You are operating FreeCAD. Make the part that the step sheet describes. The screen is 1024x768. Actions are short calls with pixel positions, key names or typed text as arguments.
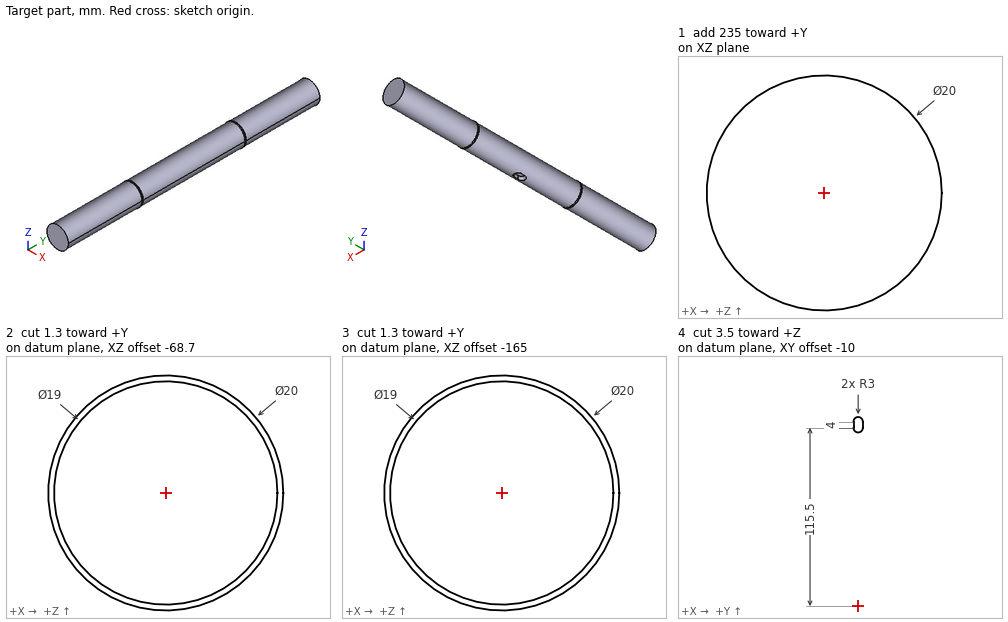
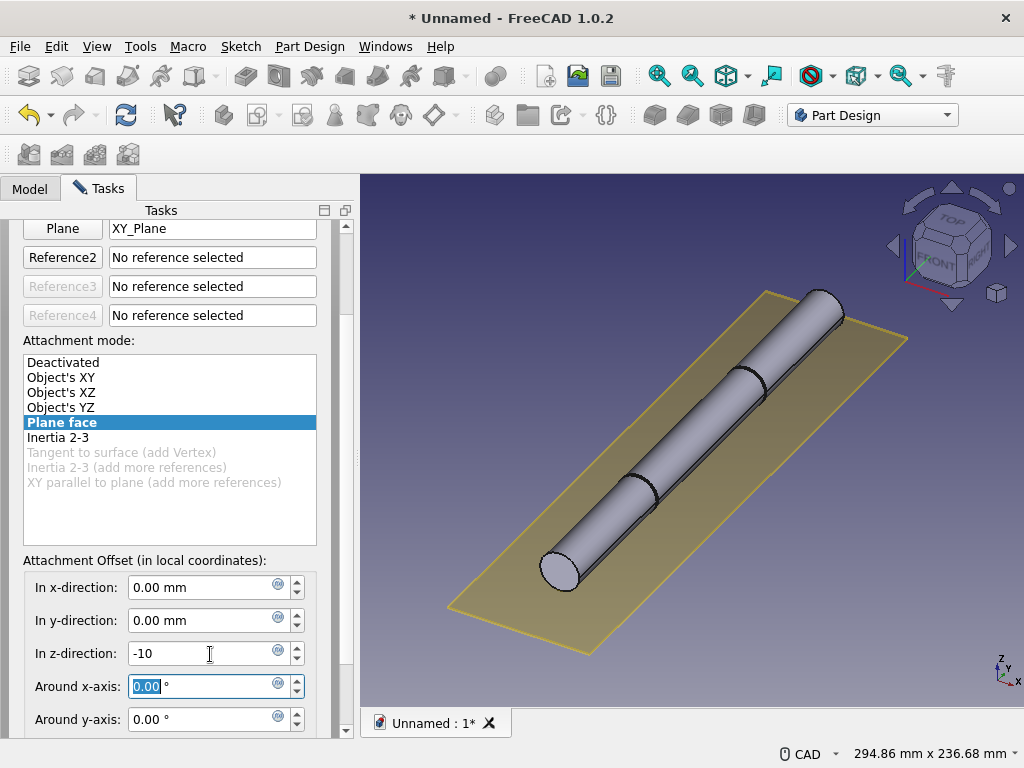
scroll(346, 479, up, 3)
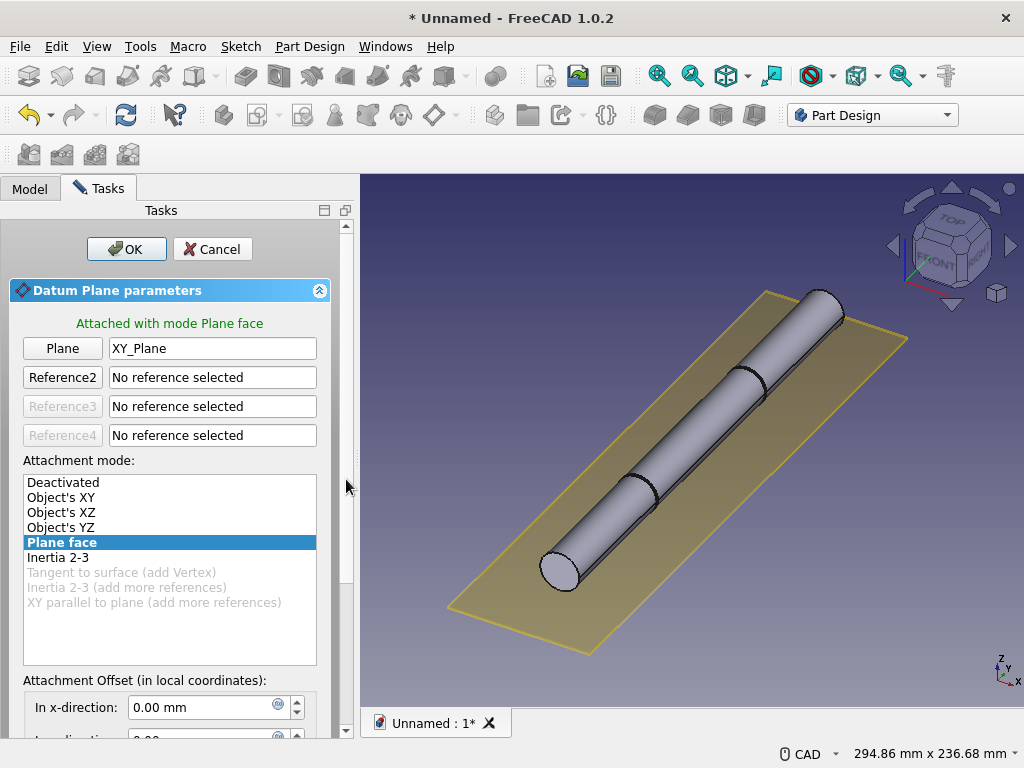
click(127, 249)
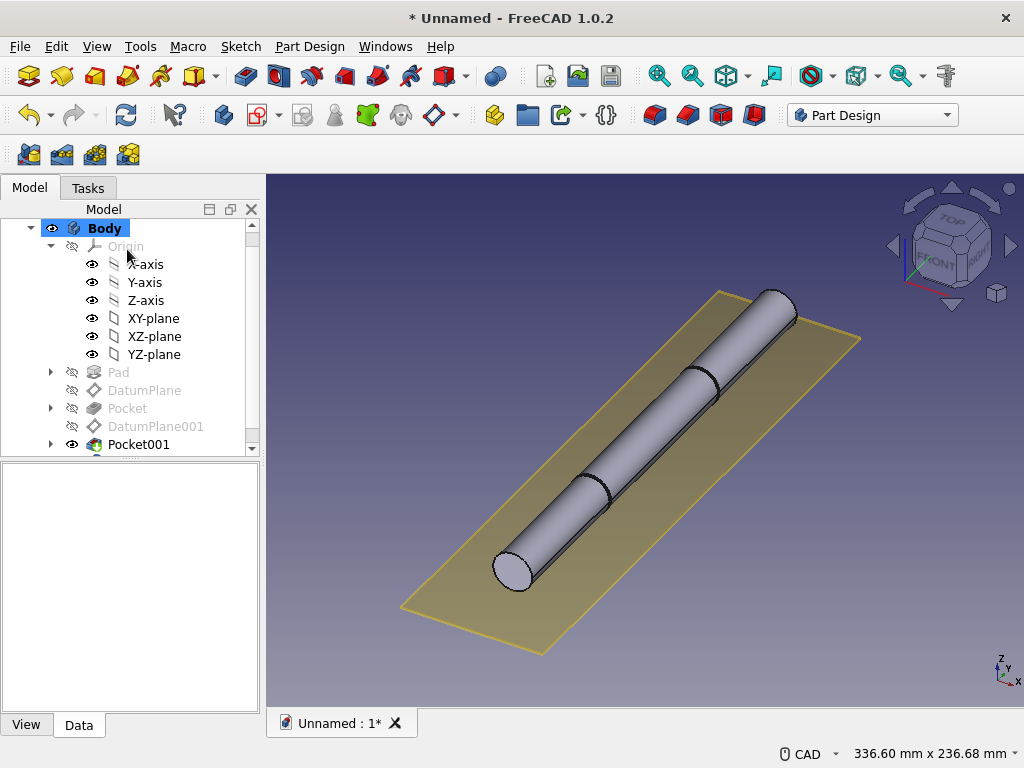
scroll(121, 332, down, 3)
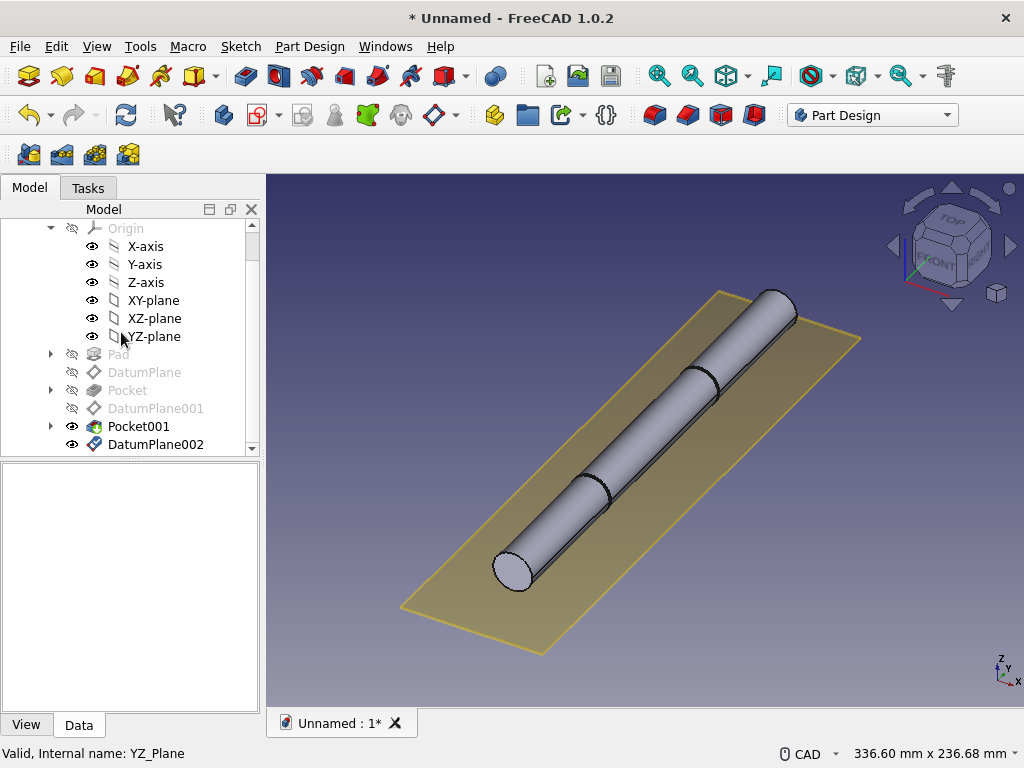
click(117, 444)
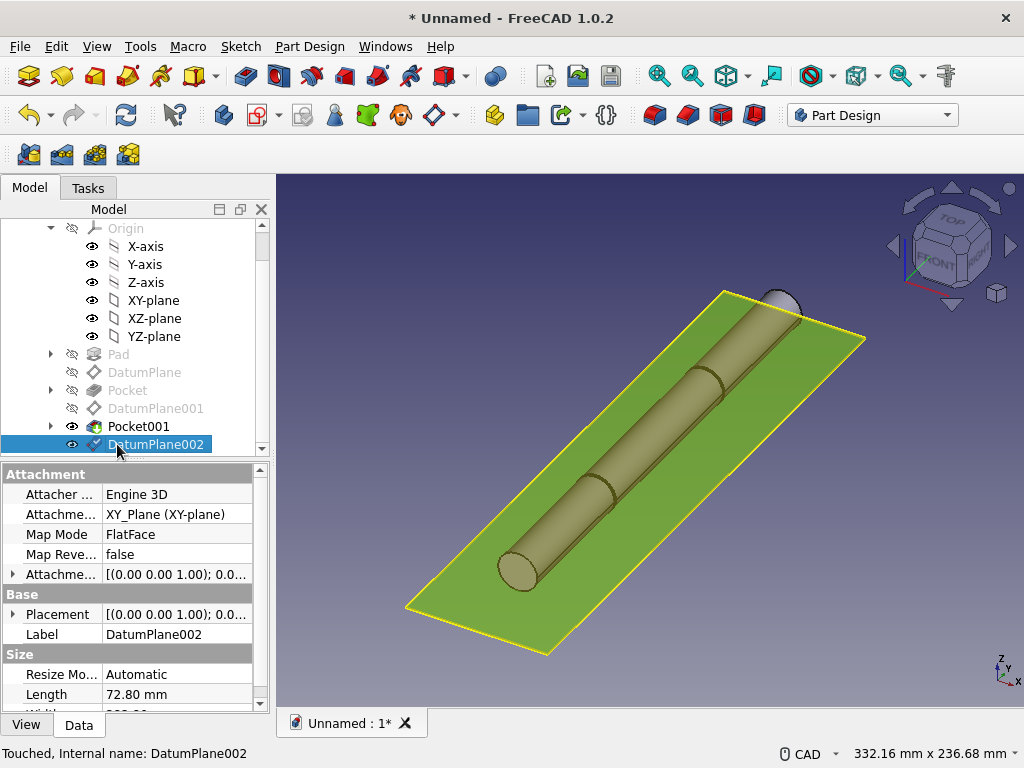
click(256, 116)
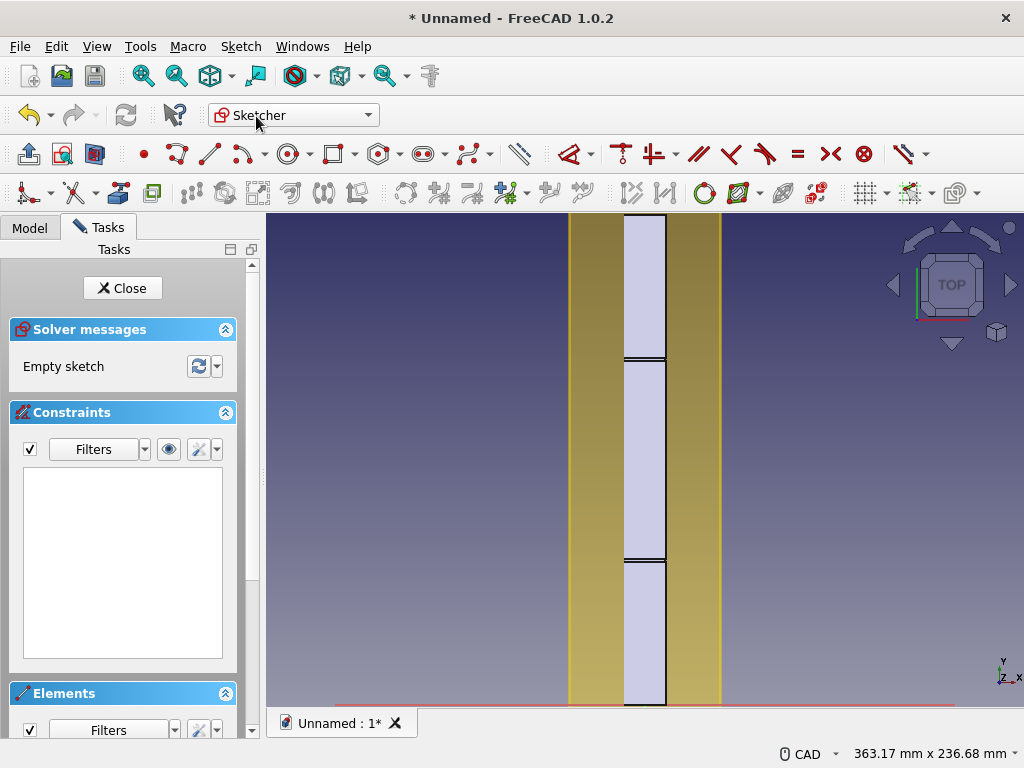
key(q)
key(s)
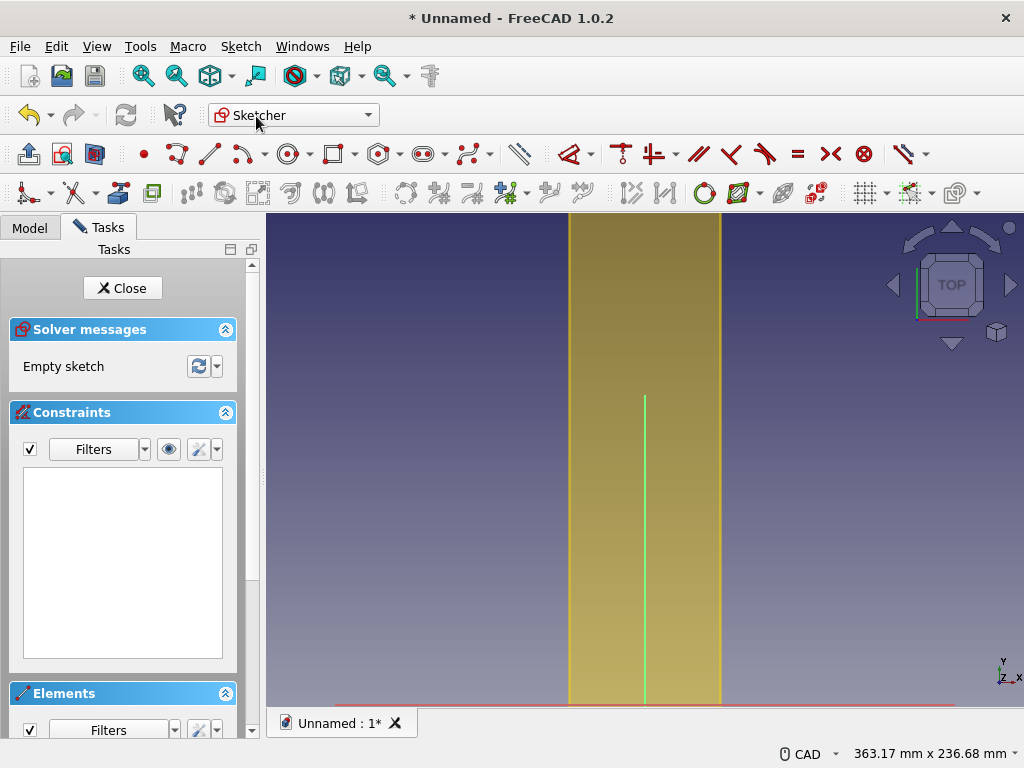
scroll(650, 460, up, 13)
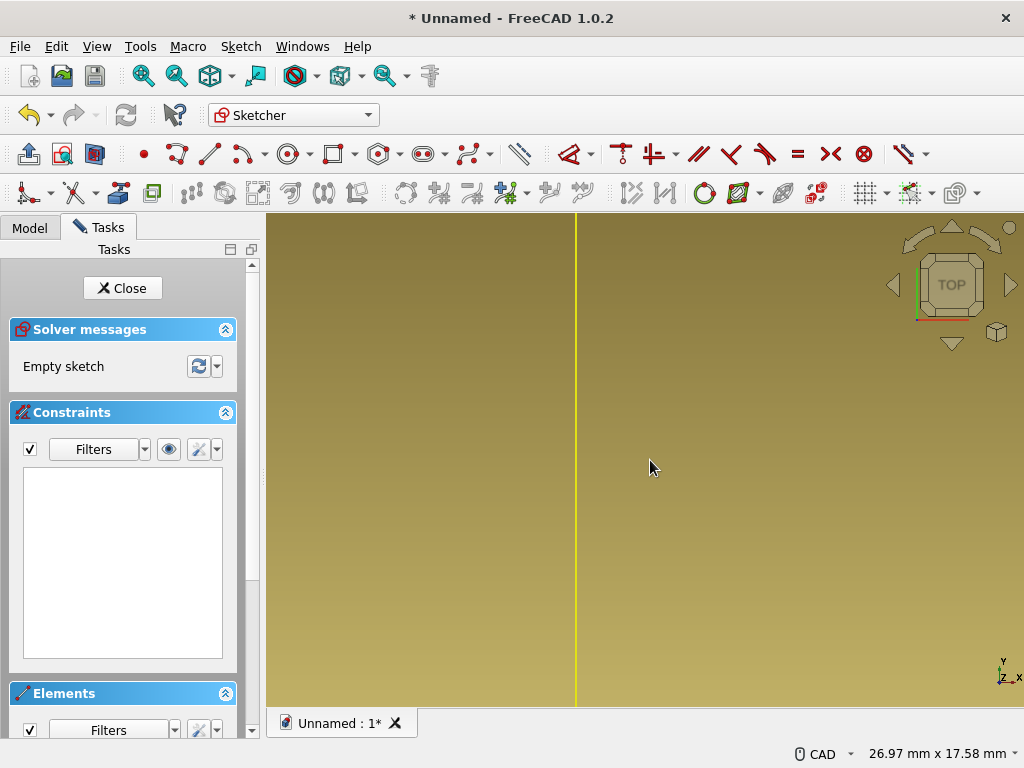
click(422, 154)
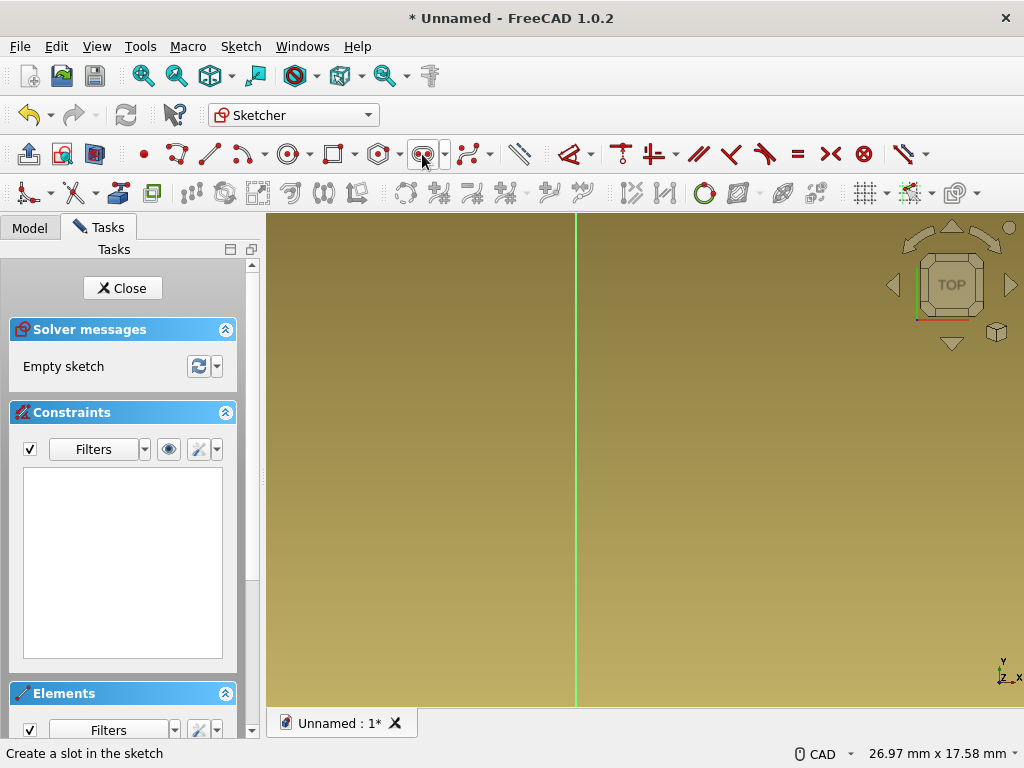
click(576, 510)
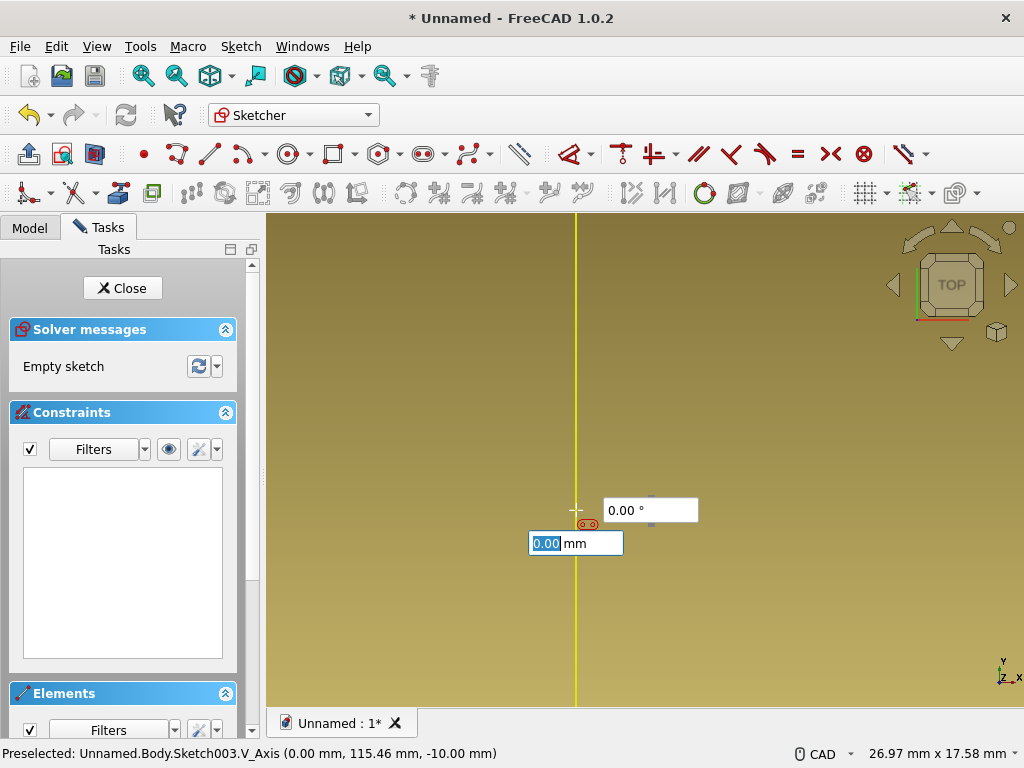
click(585, 398)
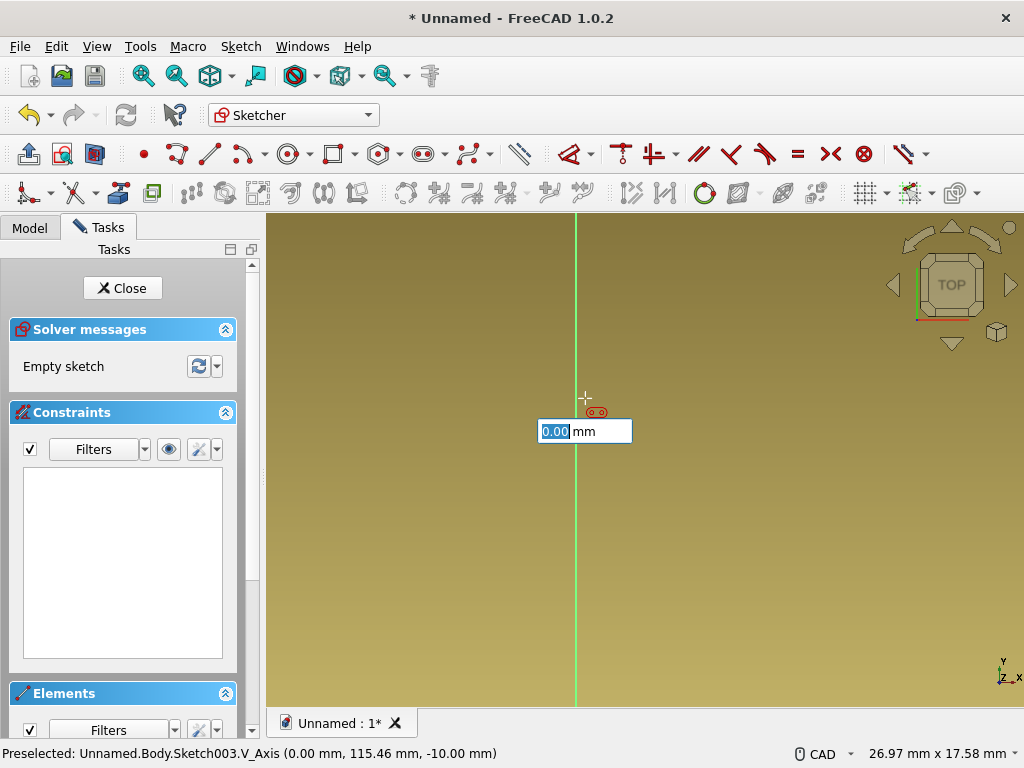
click(661, 454)
key(Escape)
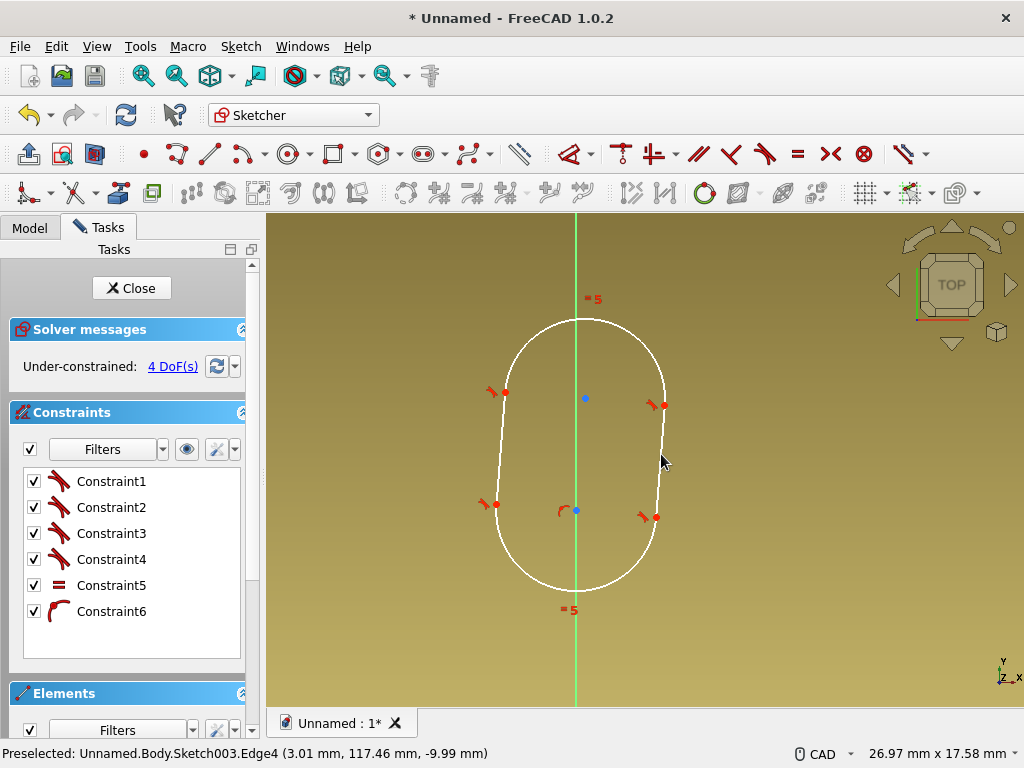
click(499, 471)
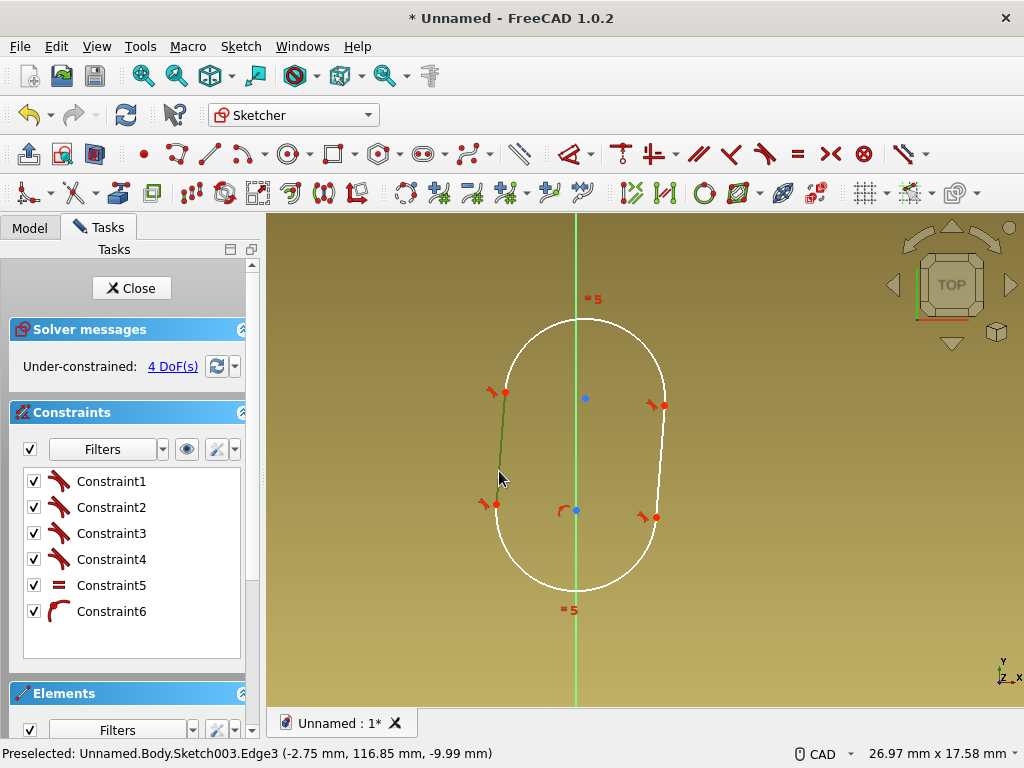
key(v)